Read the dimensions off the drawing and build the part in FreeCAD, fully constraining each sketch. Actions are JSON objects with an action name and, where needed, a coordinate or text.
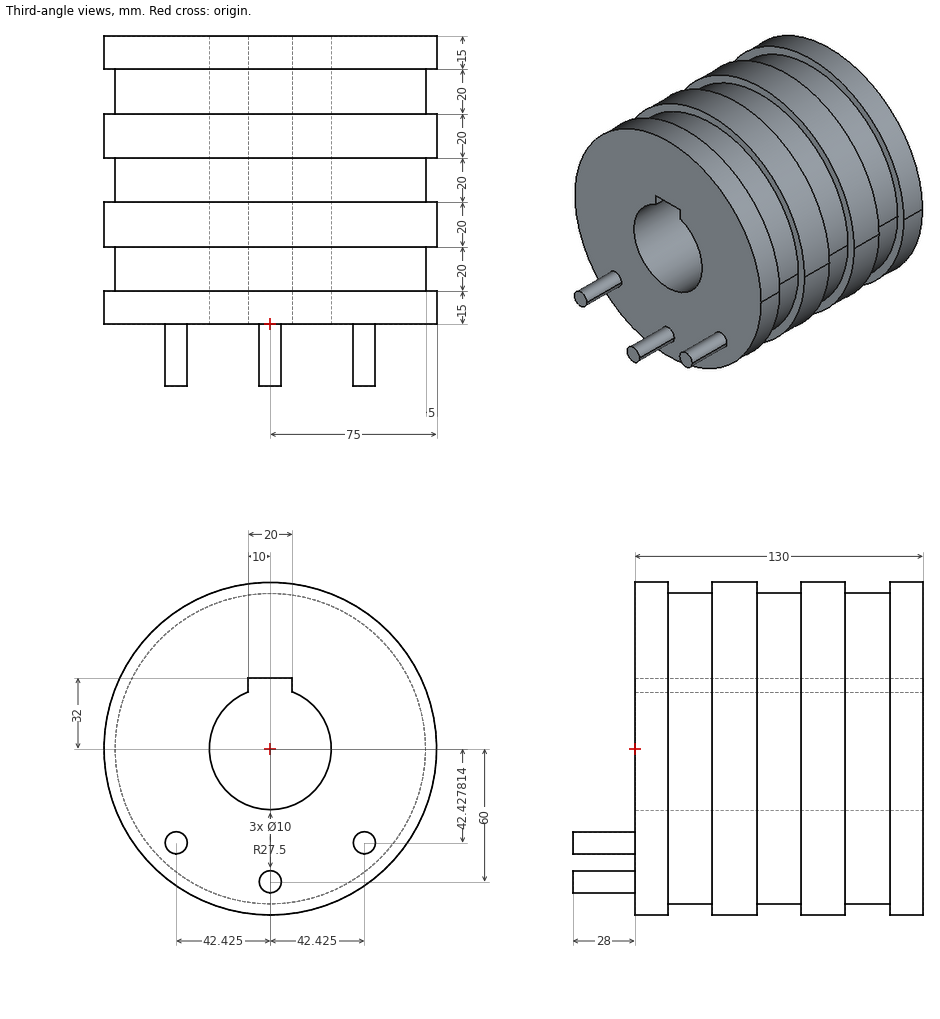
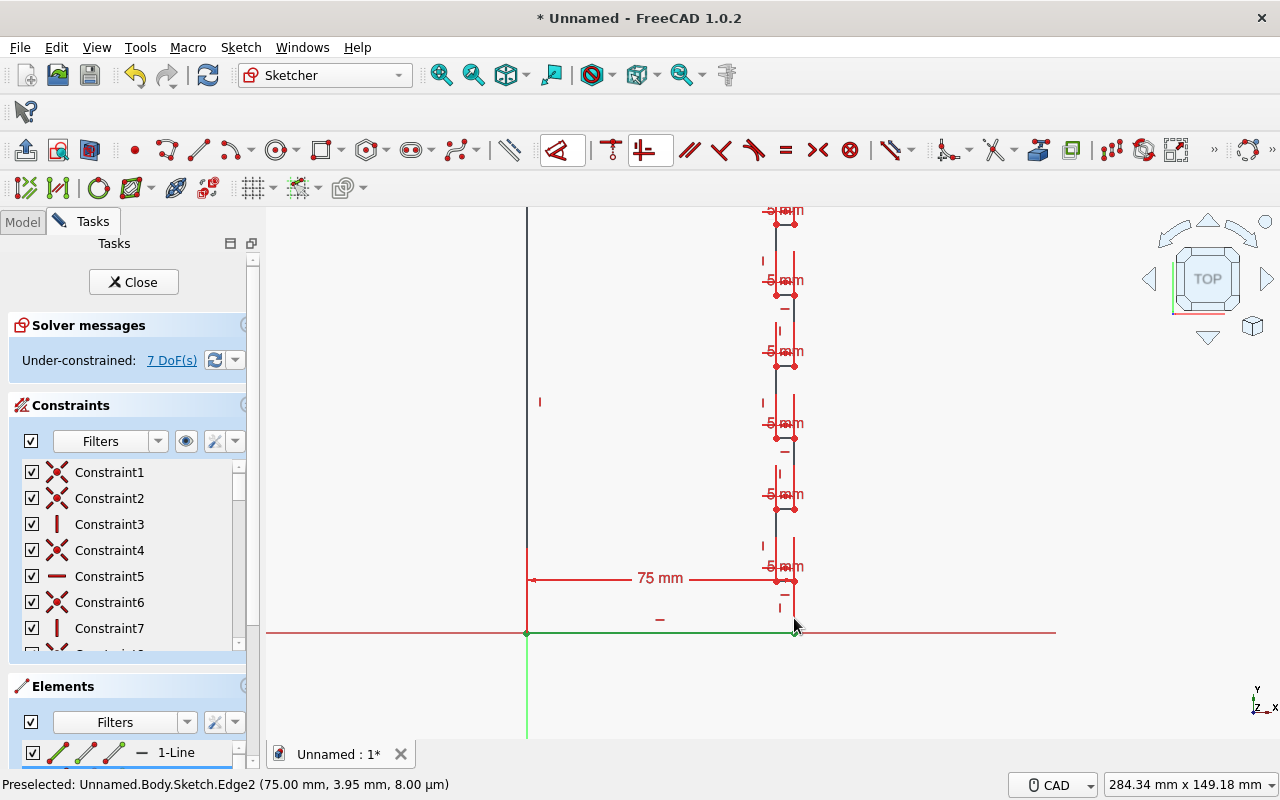
{"action": "key", "text": "i"}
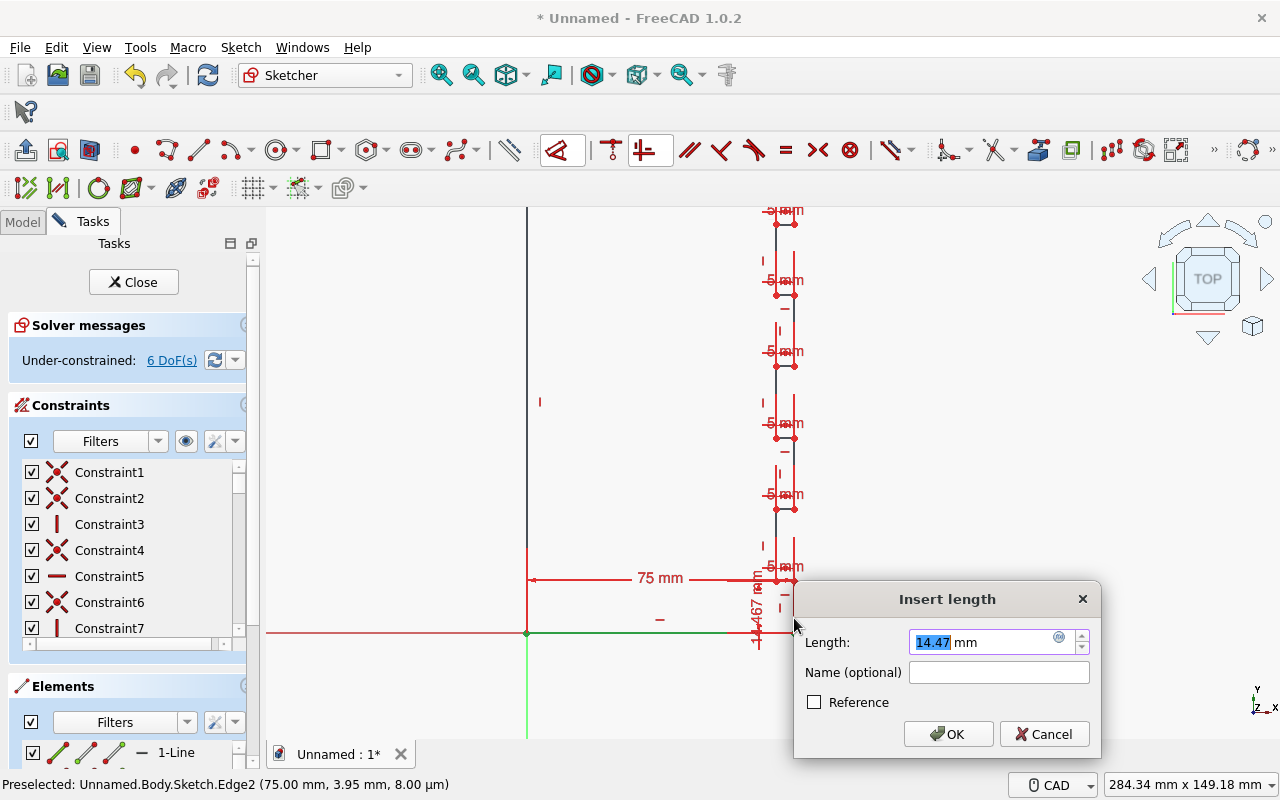
{"action": "type", "text": "15"}
{"action": "key", "text": "Return"}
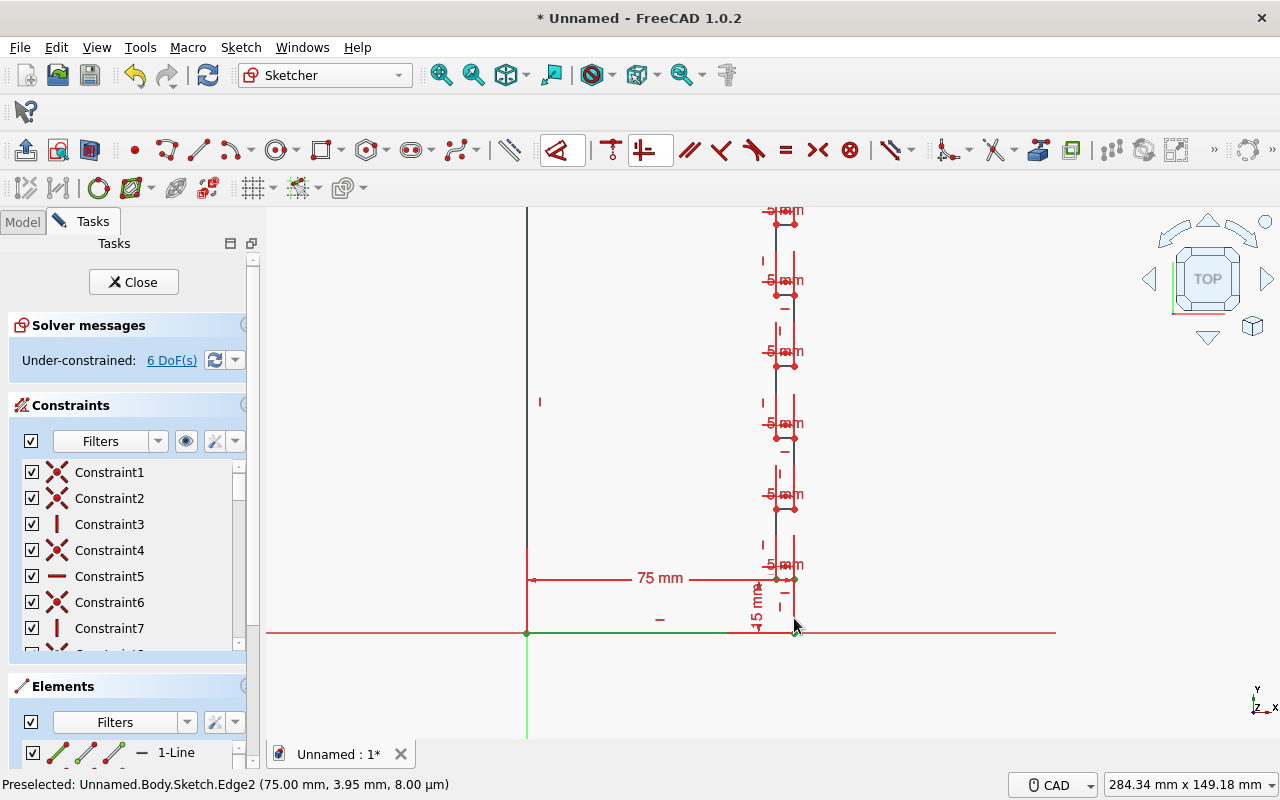
{"action": "left_click", "coordinate": [776, 530]}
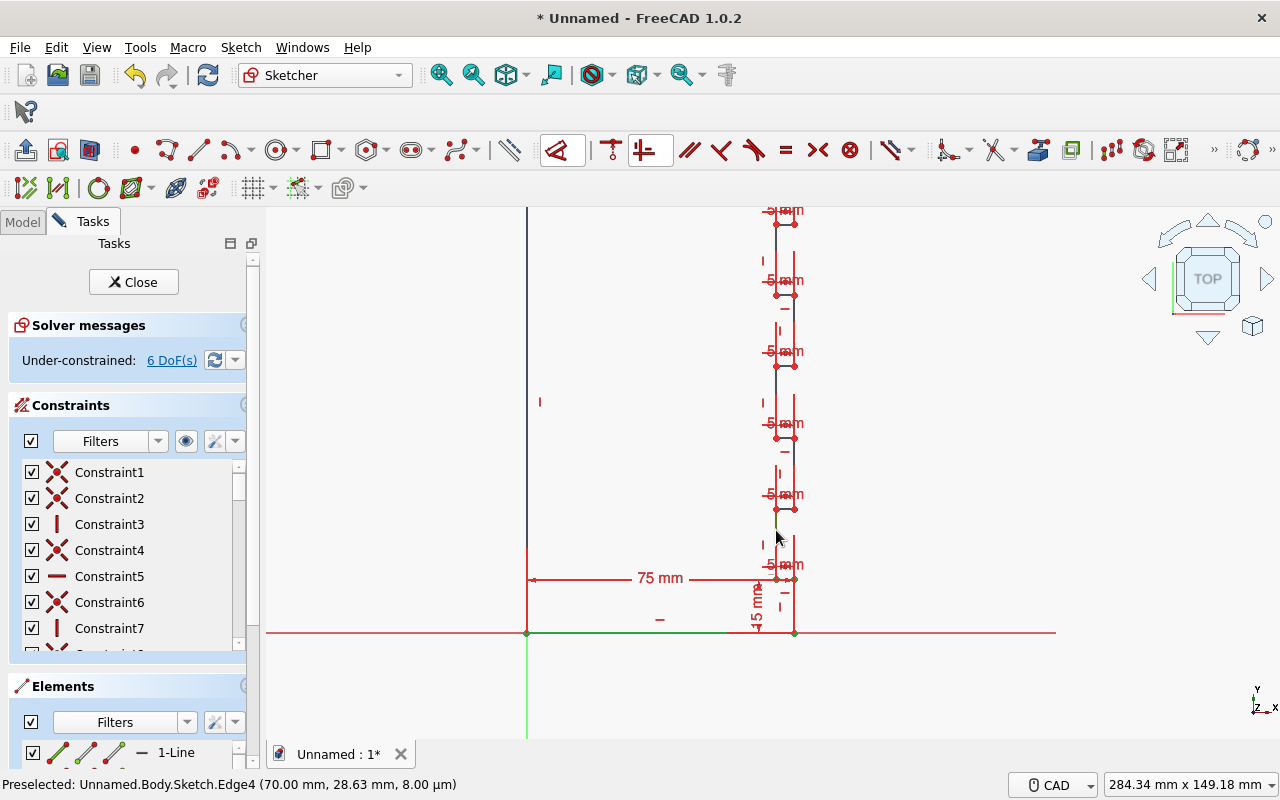
{"action": "key", "text": "i"}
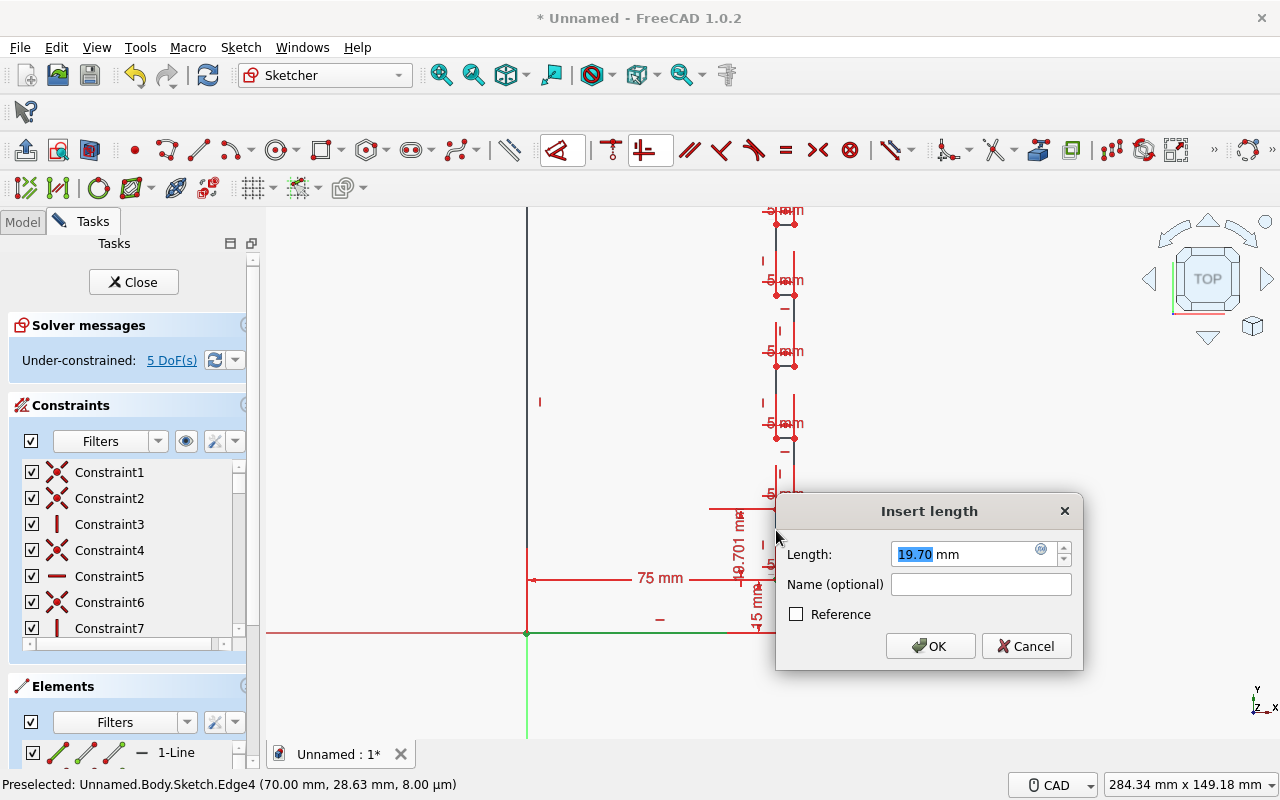
{"action": "type", "text": "20"}
{"action": "key", "text": "Return"}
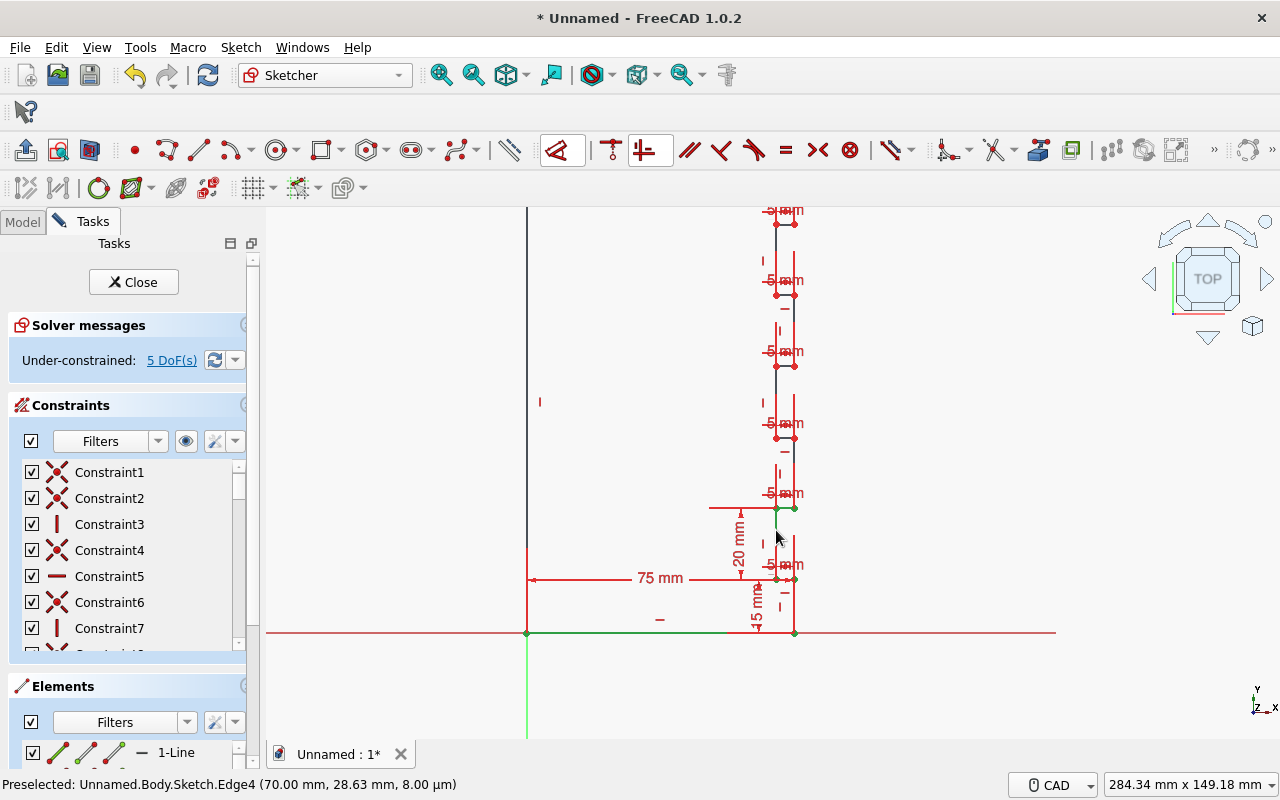
{"action": "left_click", "coordinate": [794, 459]}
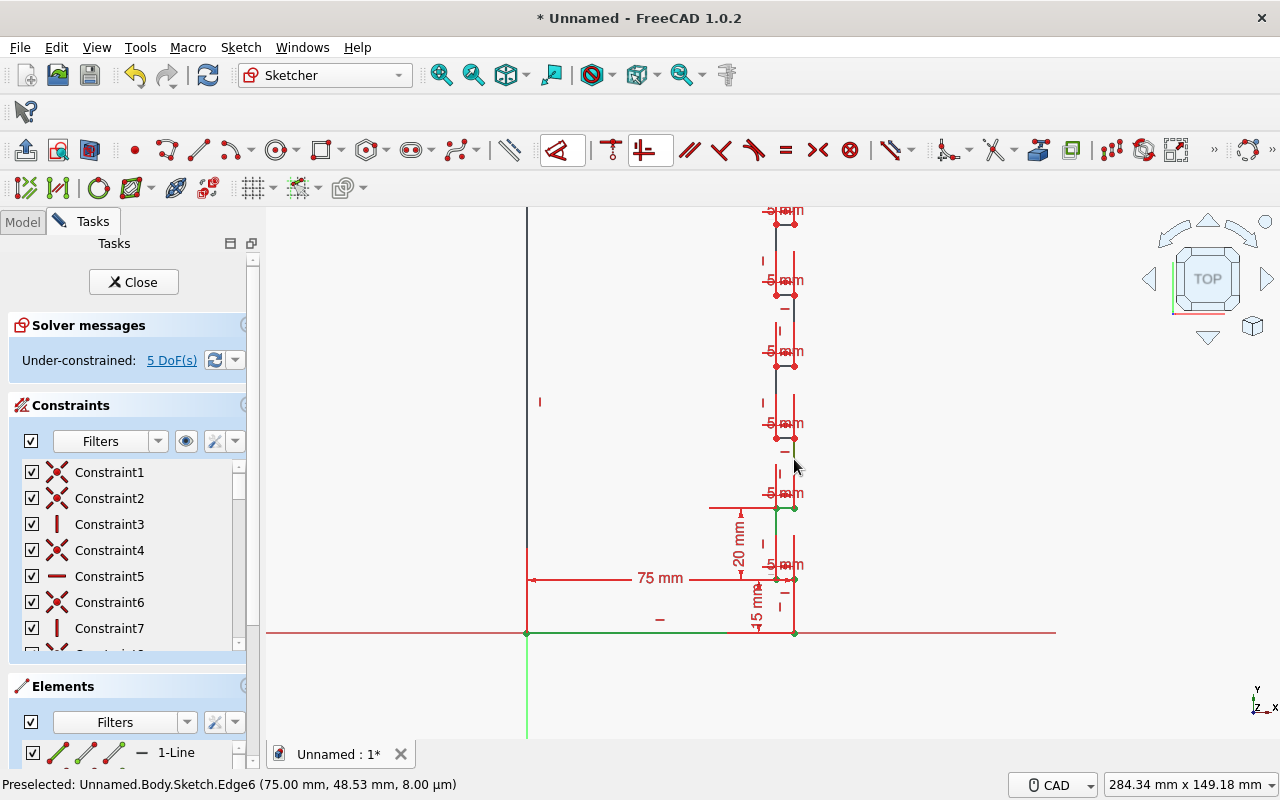
{"action": "key", "text": "i"}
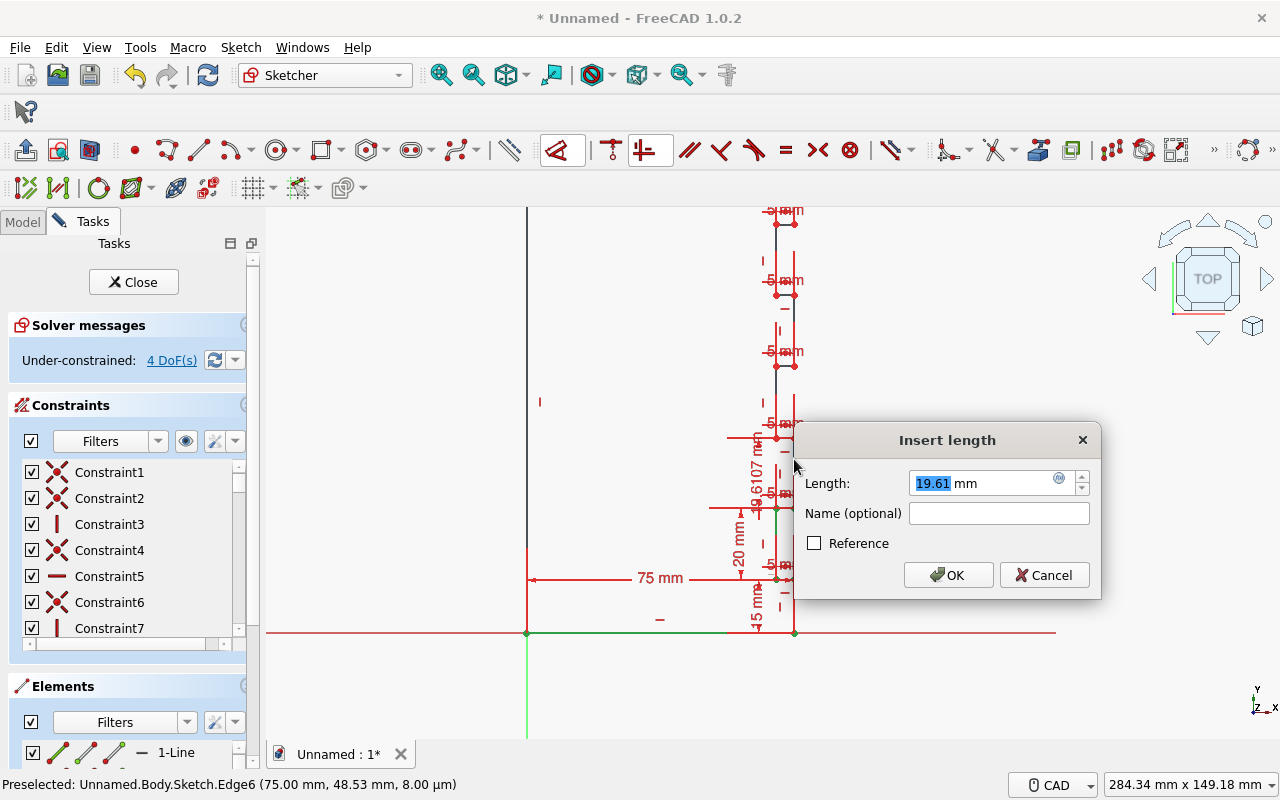
{"action": "type", "text": "20"}
{"action": "key", "text": "Return"}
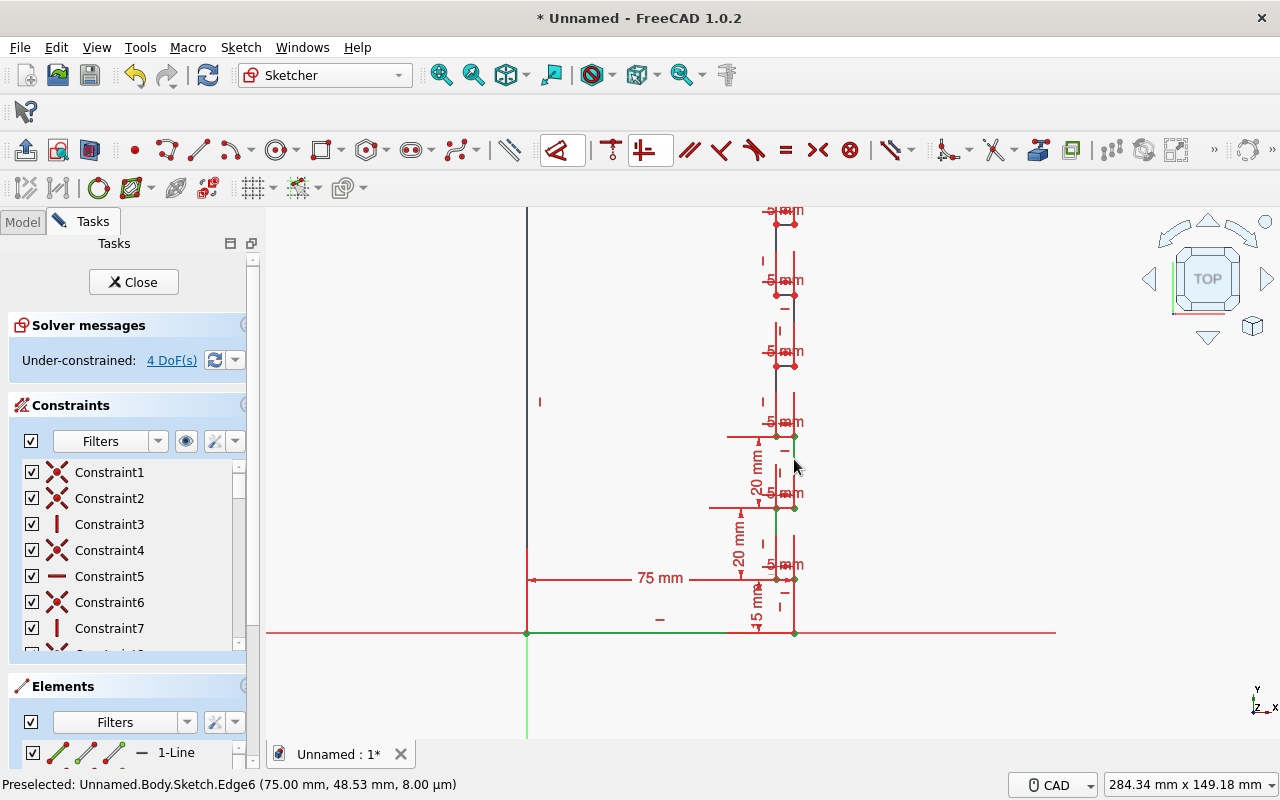
{"action": "left_click", "coordinate": [776, 388]}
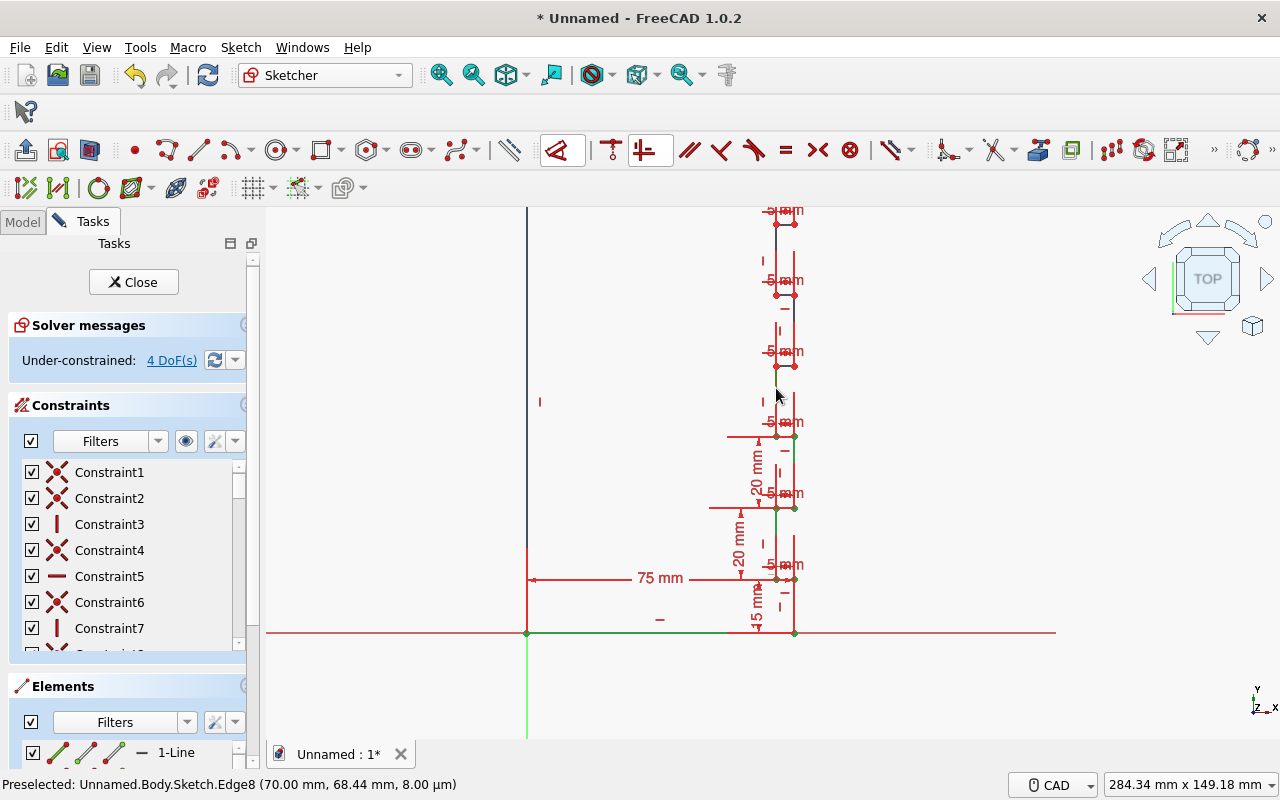
{"action": "key", "text": "i"}